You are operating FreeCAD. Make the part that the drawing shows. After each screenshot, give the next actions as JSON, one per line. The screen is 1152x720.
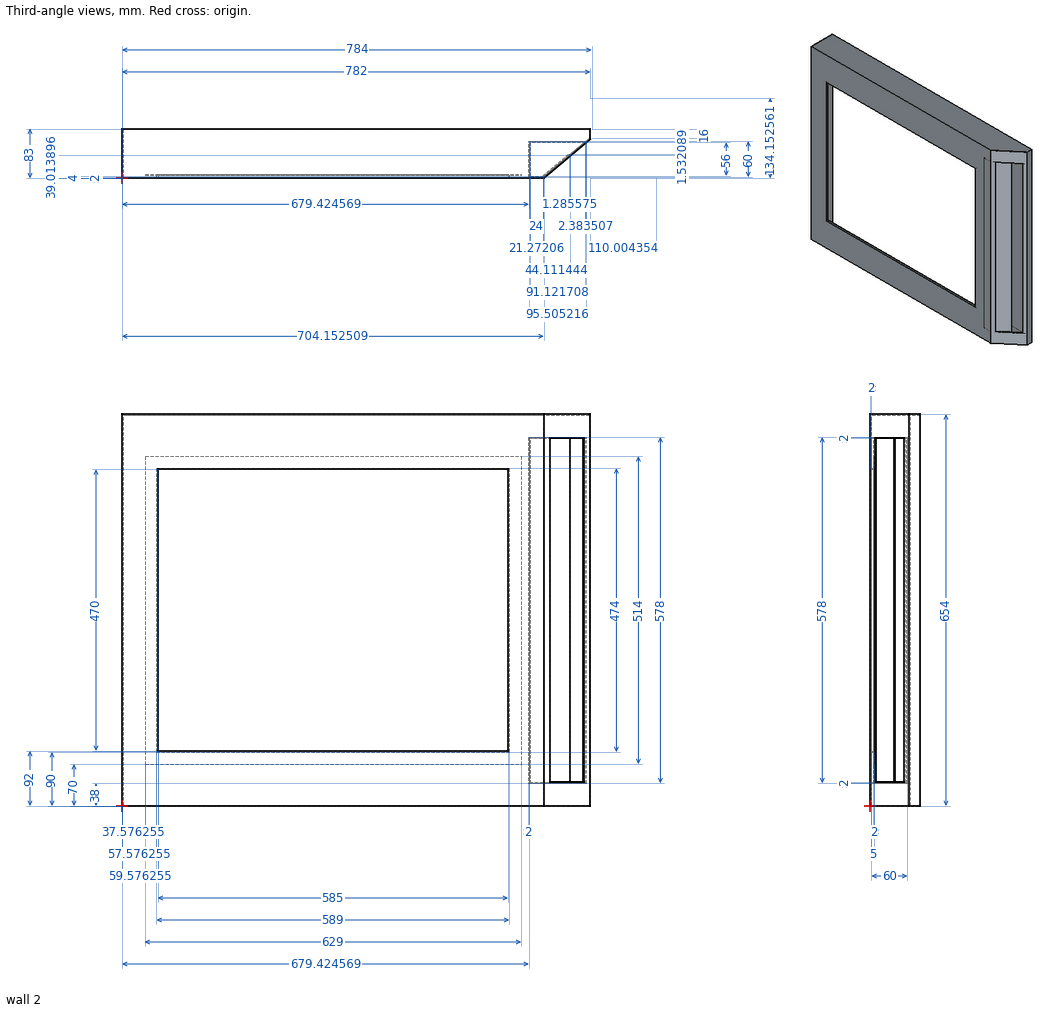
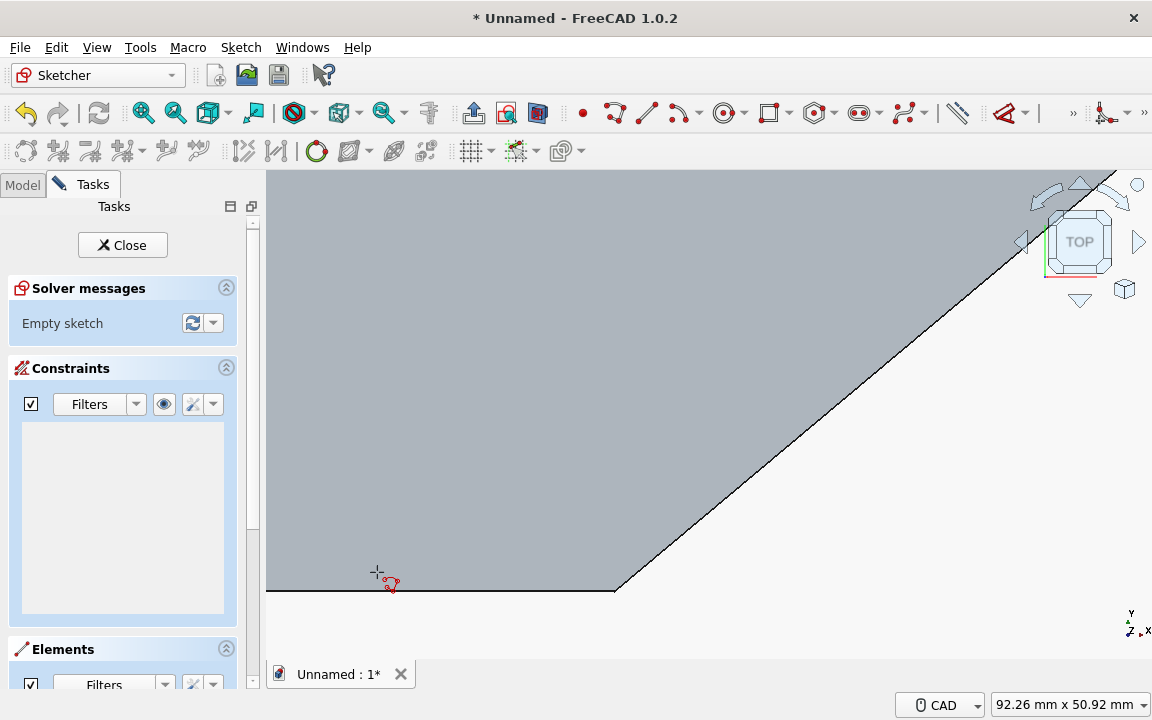
{"action": "scroll", "coordinate": [403, 573], "scroll_direction": "down", "scroll_amount": 3}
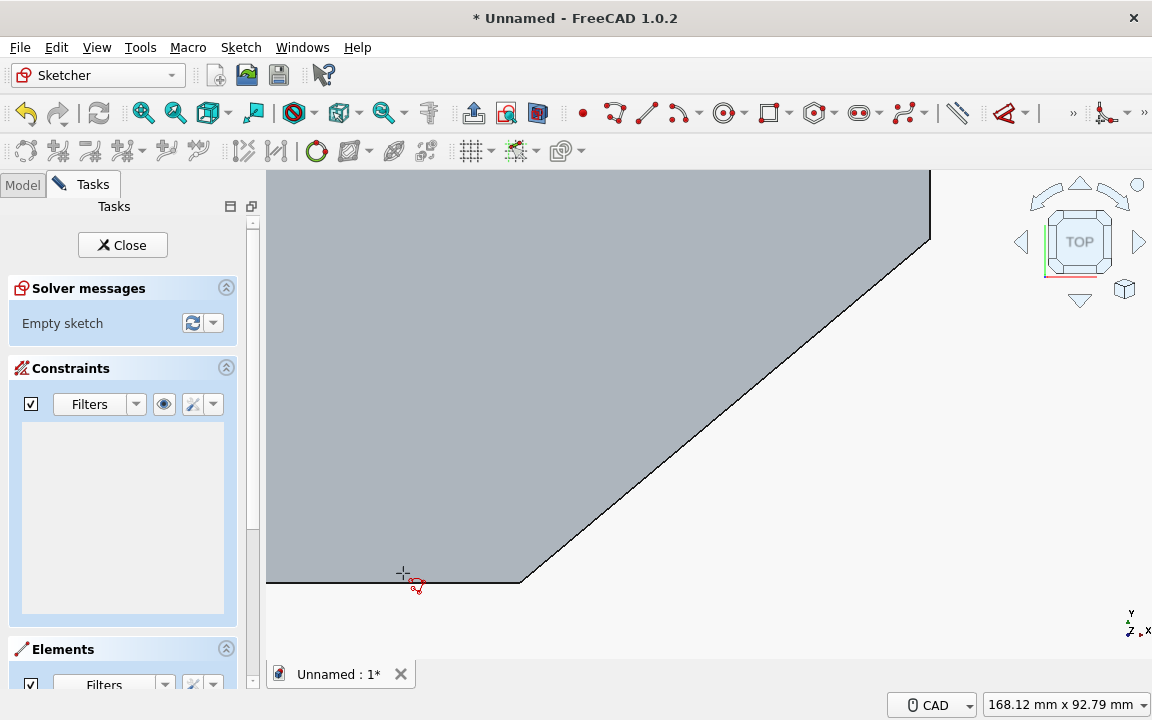
{"action": "left_click", "coordinate": [389, 257]}
{"action": "left_click", "coordinate": [892, 257]}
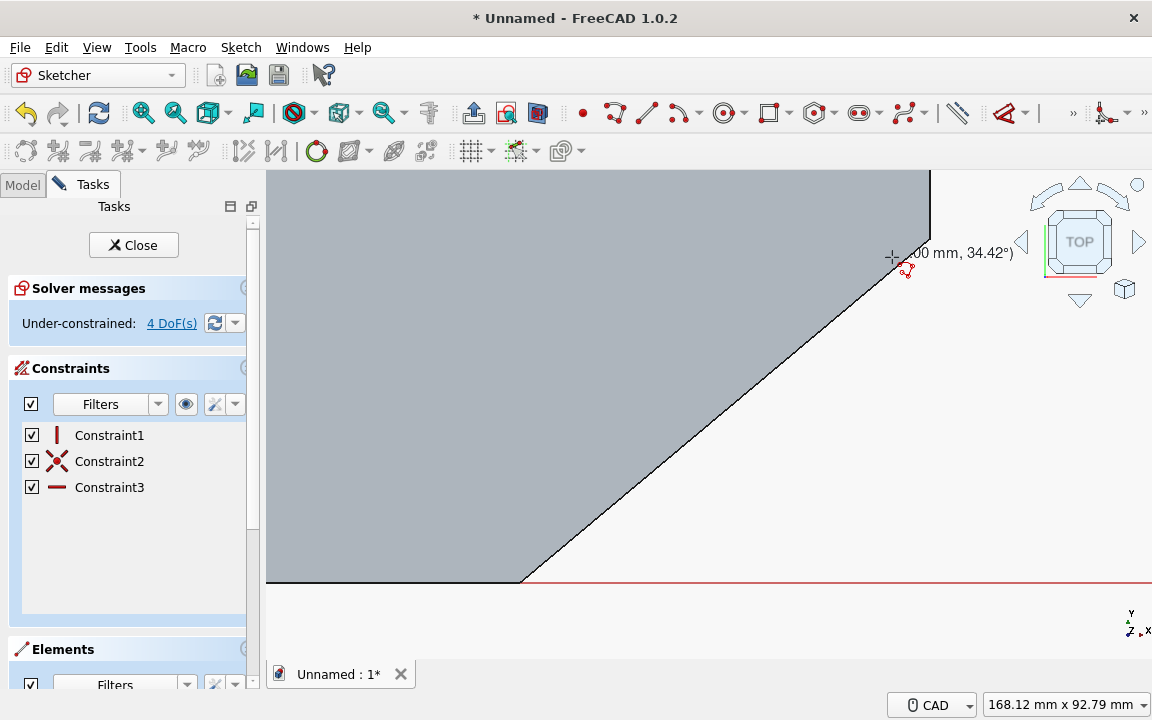
{"action": "scroll", "coordinate": [515, 573], "scroll_direction": "up", "scroll_amount": 3}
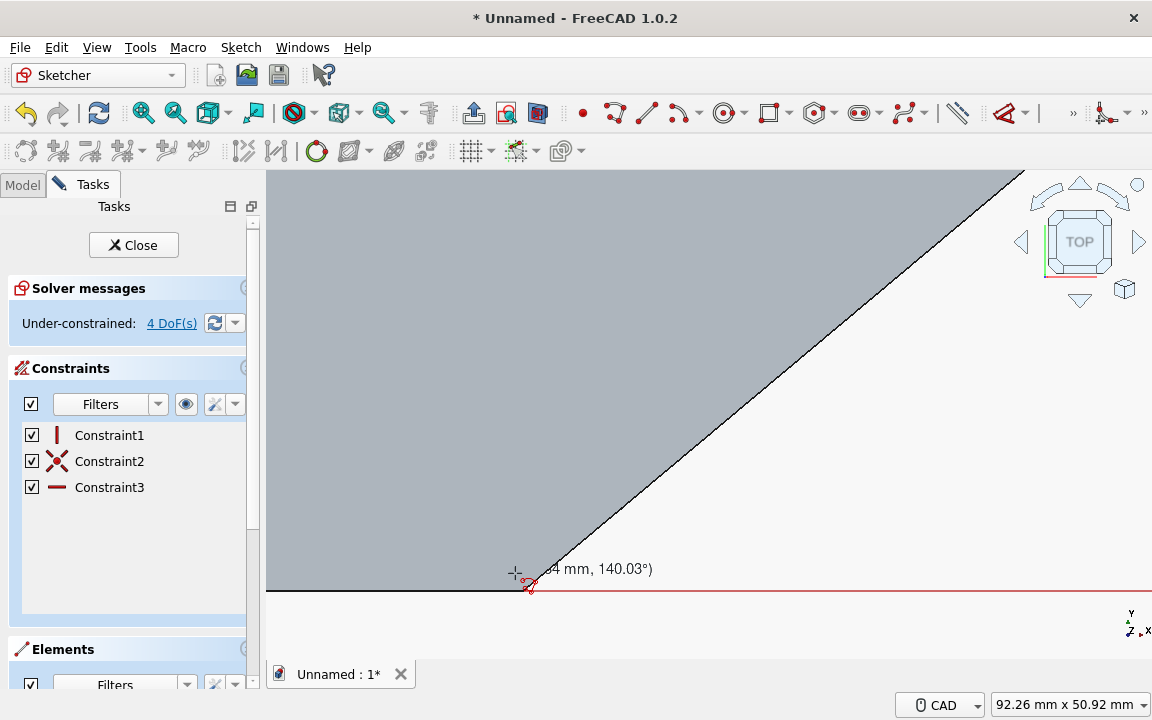
{"action": "left_click", "coordinate": [516, 572]}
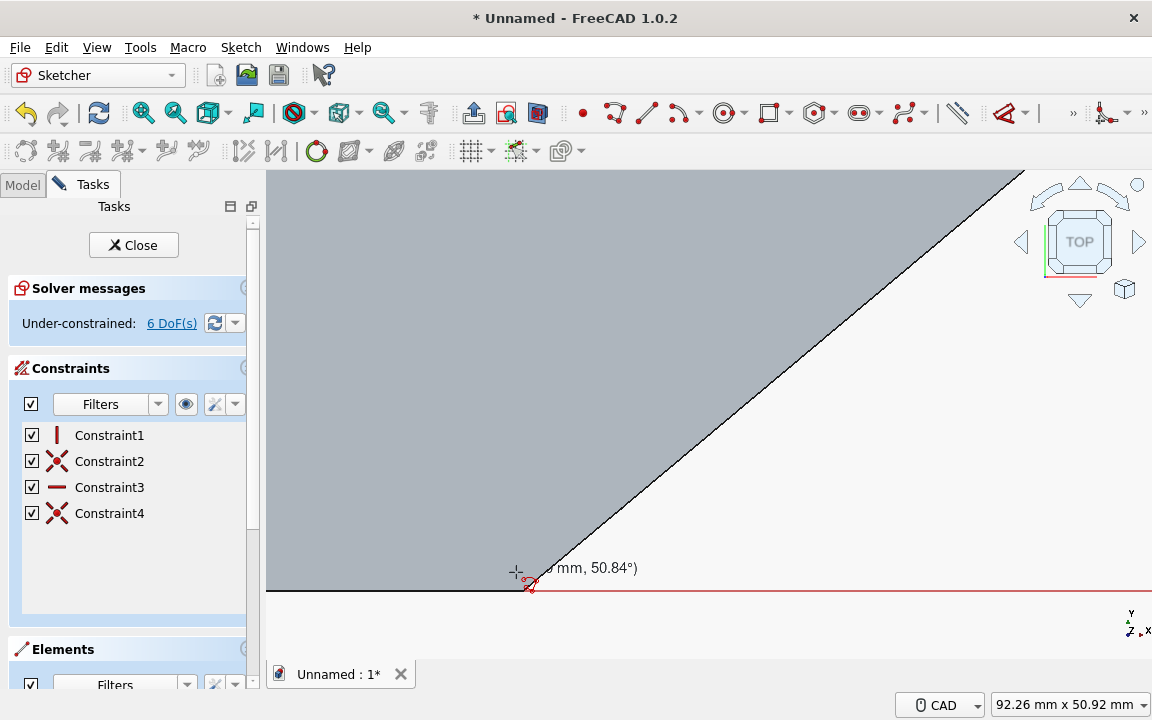
{"action": "scroll", "coordinate": [515, 573], "scroll_direction": "down", "scroll_amount": 3}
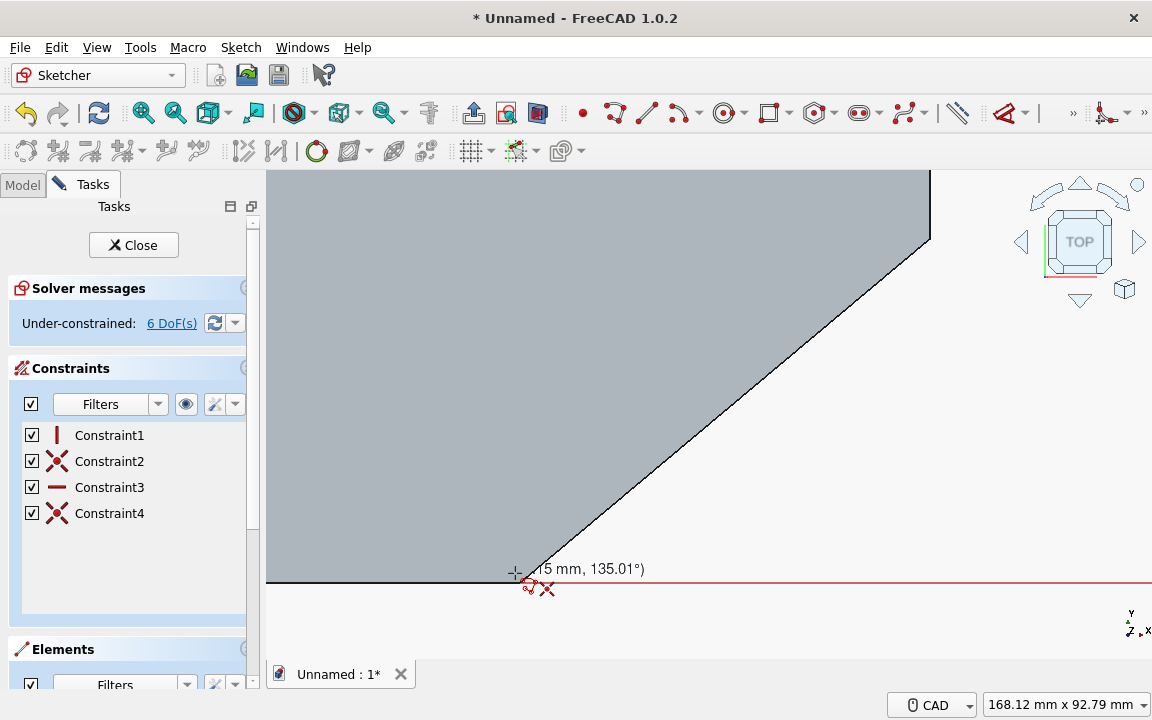
{"action": "scroll", "coordinate": [389, 573], "scroll_direction": "up", "scroll_amount": 3}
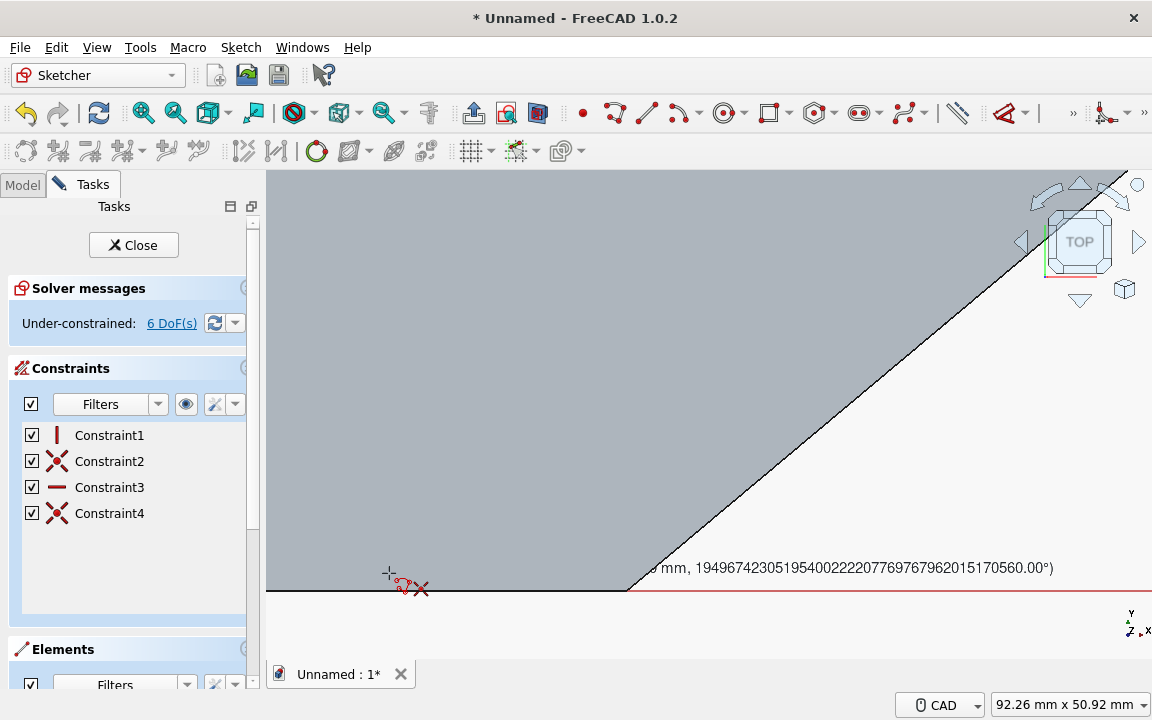
{"action": "left_click", "coordinate": [389, 573]}
{"action": "key", "text": "Escape"}
{"action": "key", "text": "Escape"}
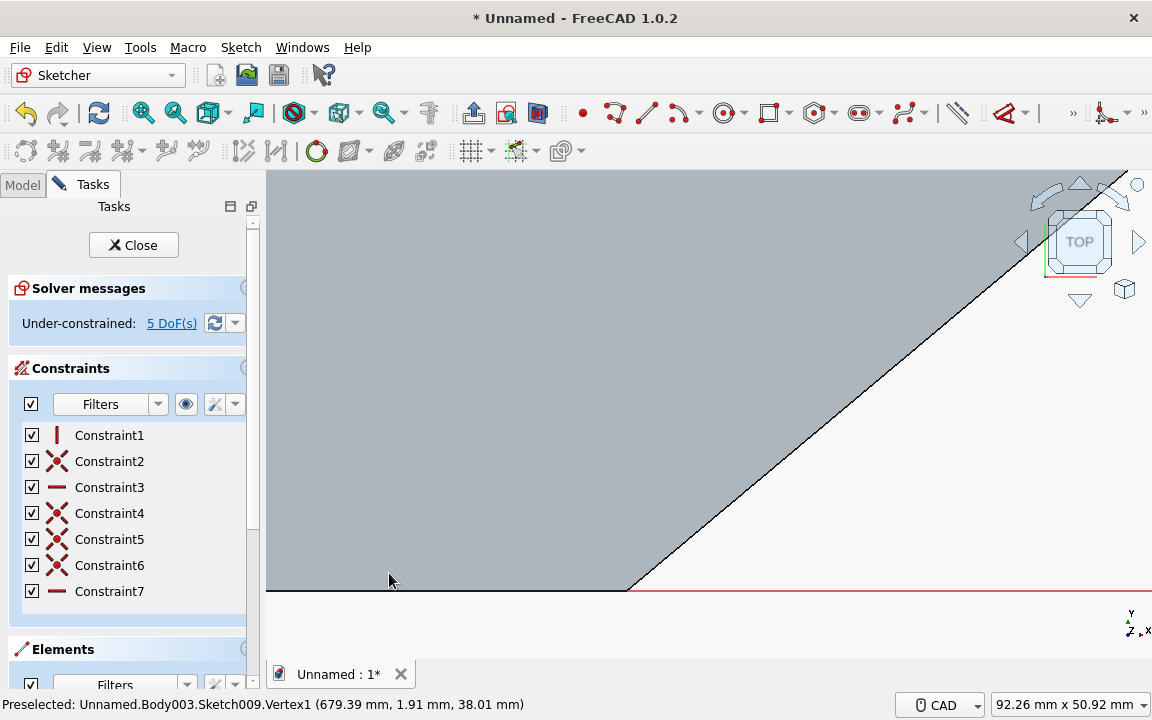
{"action": "key", "text": "d"}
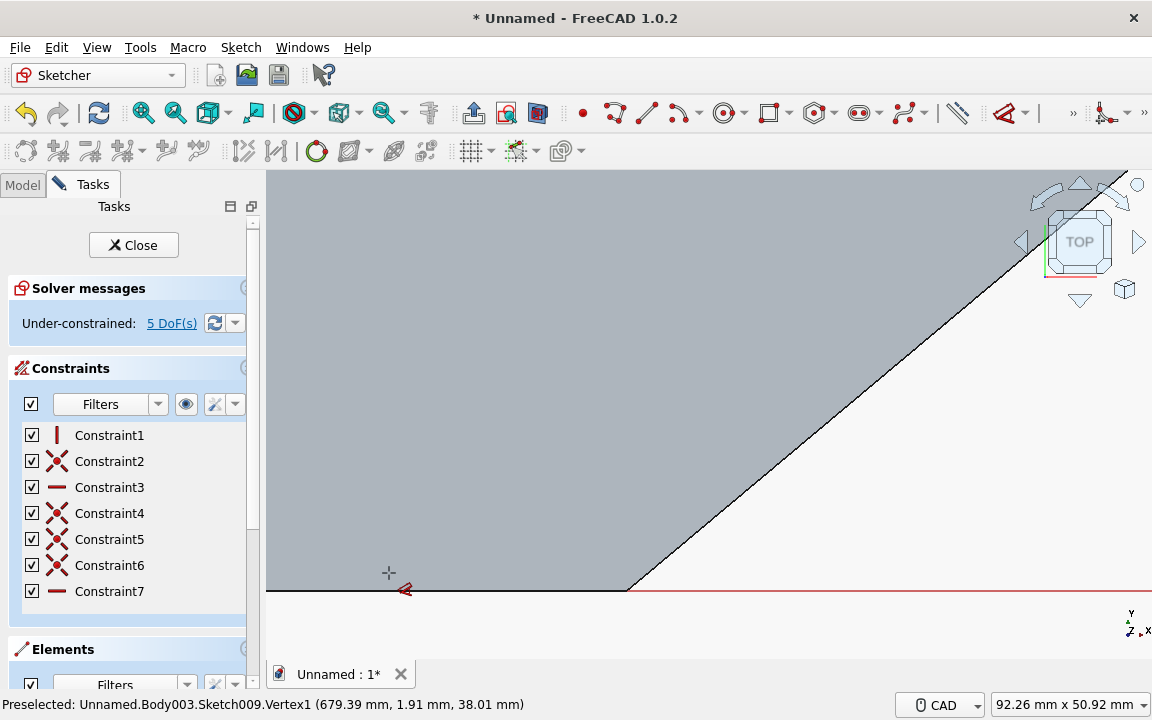
{"action": "left_click", "coordinate": [389, 401]}
{"action": "left_click", "coordinate": [355, 386]}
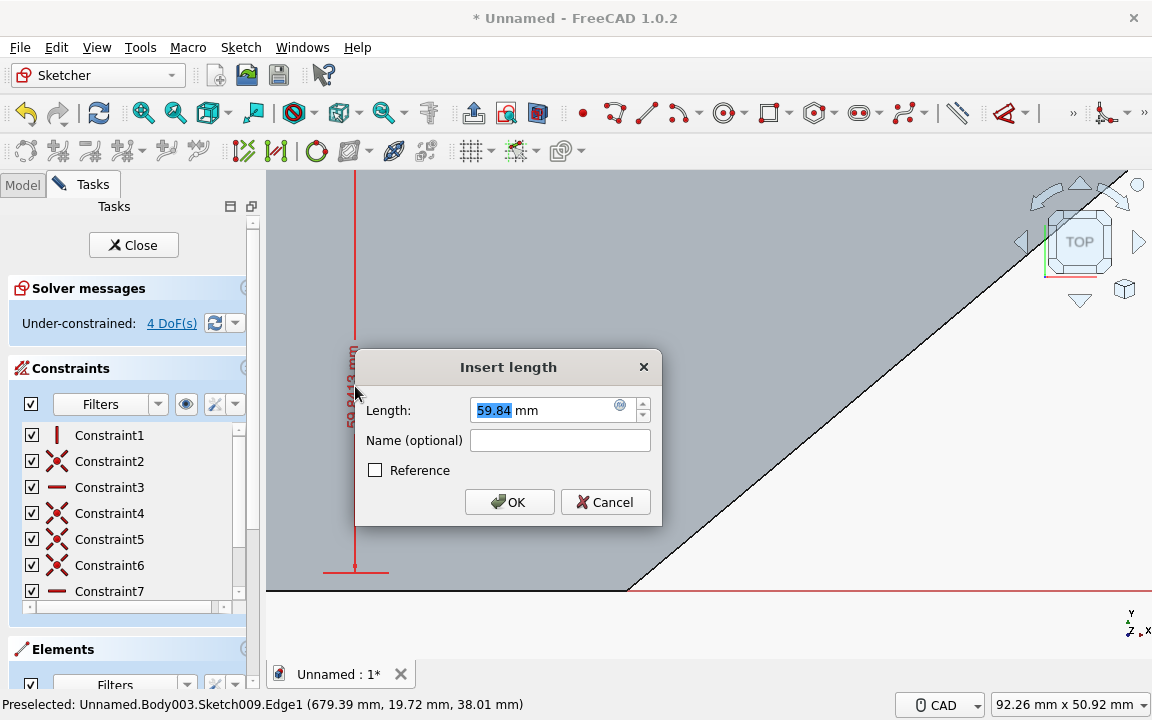
{"action": "type", "text": "60"}
{"action": "key", "text": "Return"}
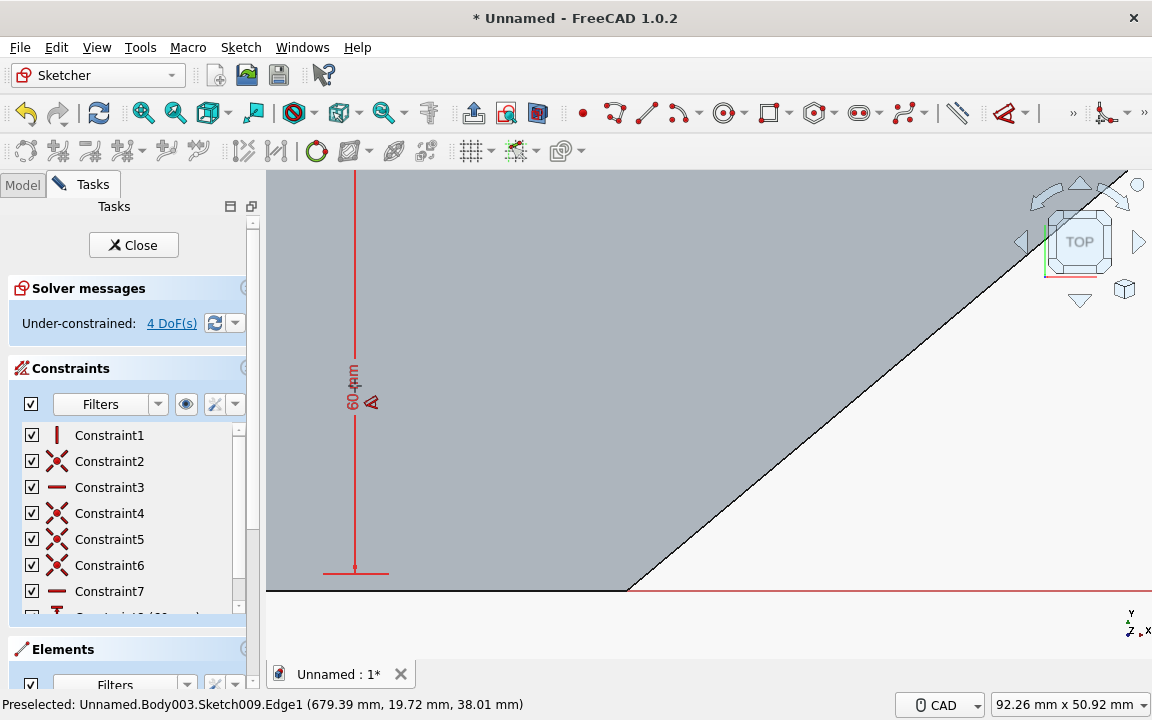
{"action": "left_click", "coordinate": [550, 574]}
{"action": "left_click", "coordinate": [504, 608]}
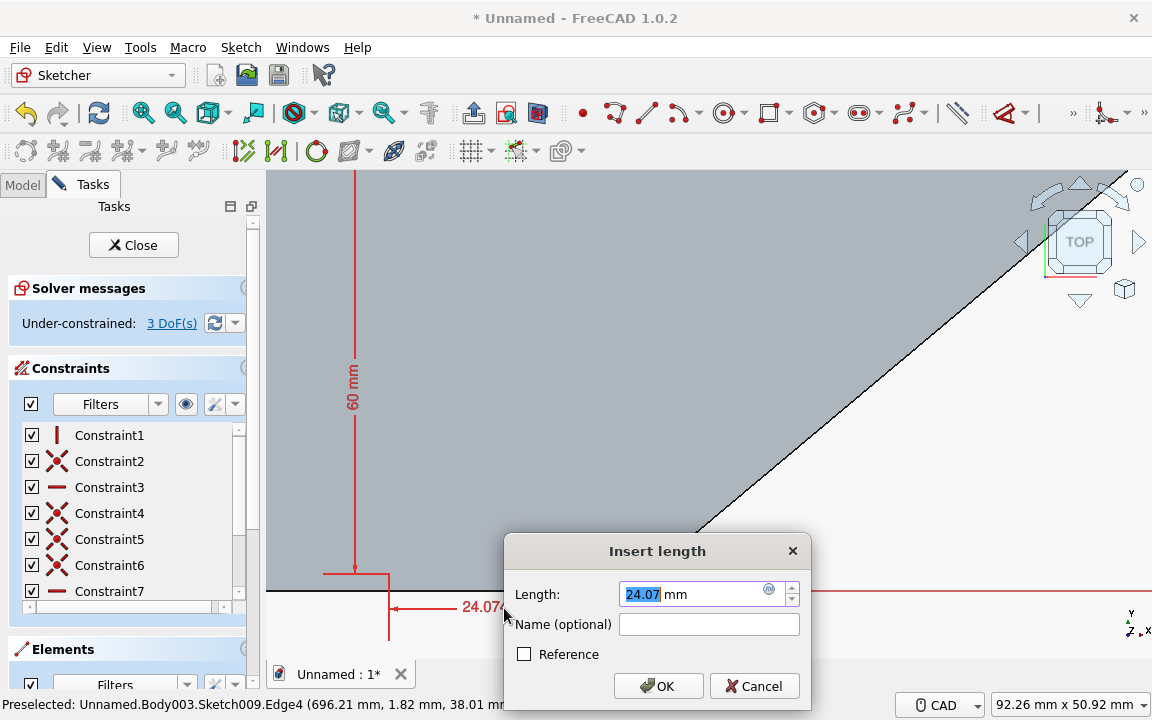
{"action": "type", "text": "24"}
{"action": "key", "text": "Return"}